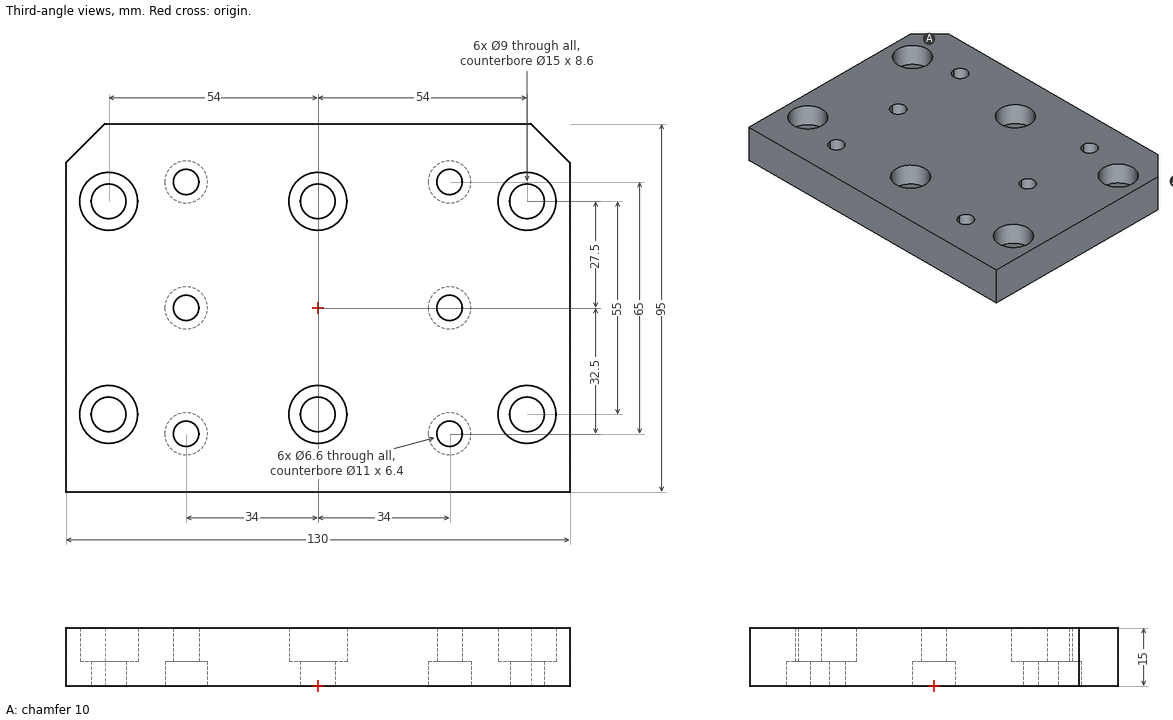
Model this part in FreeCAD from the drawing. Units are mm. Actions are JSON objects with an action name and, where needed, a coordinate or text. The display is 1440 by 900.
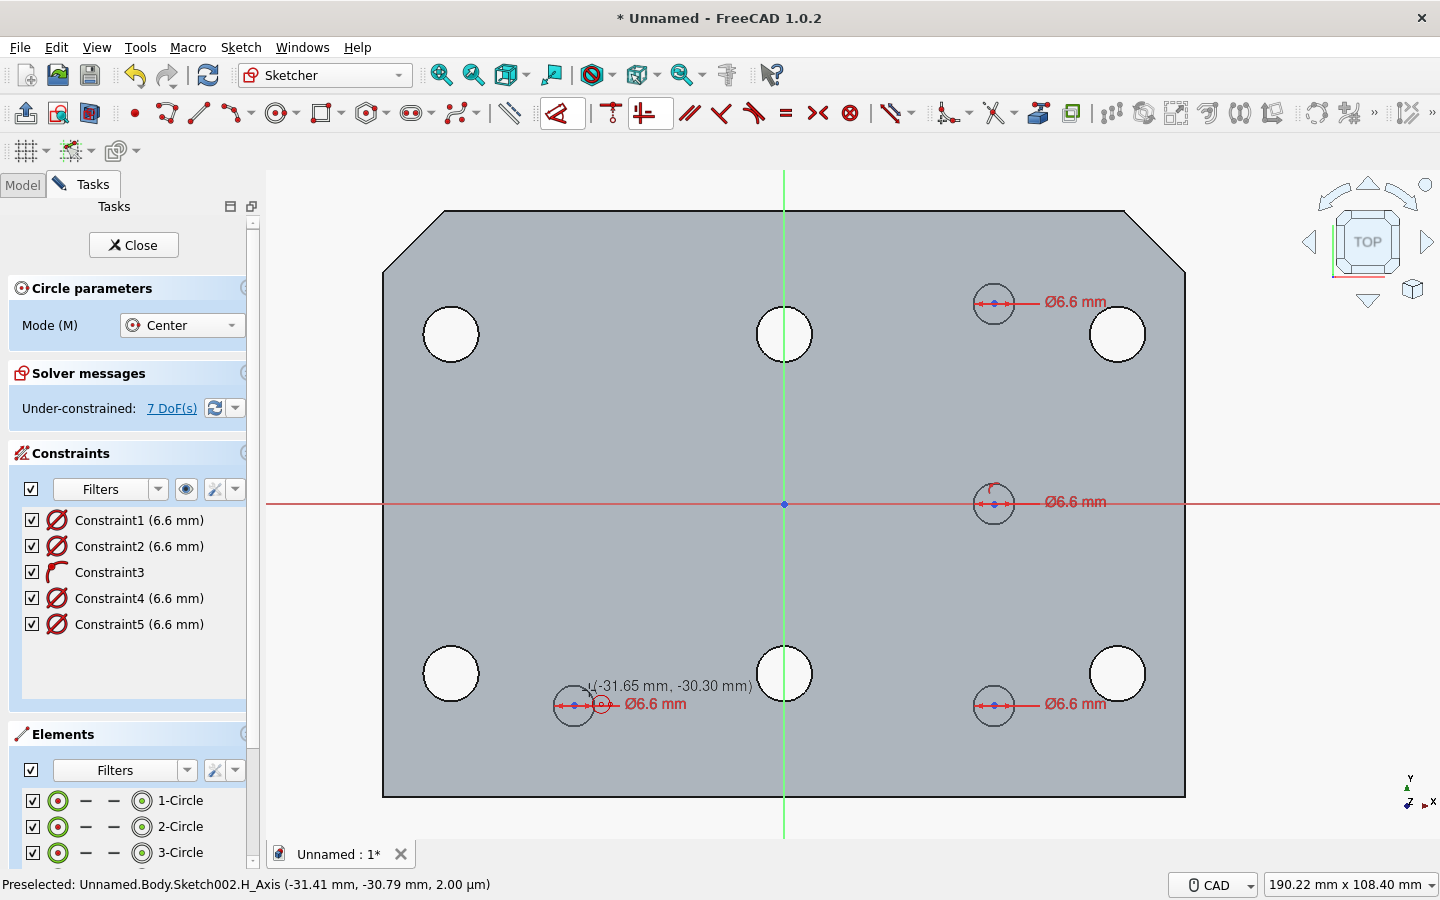
{"action": "left_click", "coordinate": [574, 504]}
{"action": "mouse_move", "coordinate": [589, 490]}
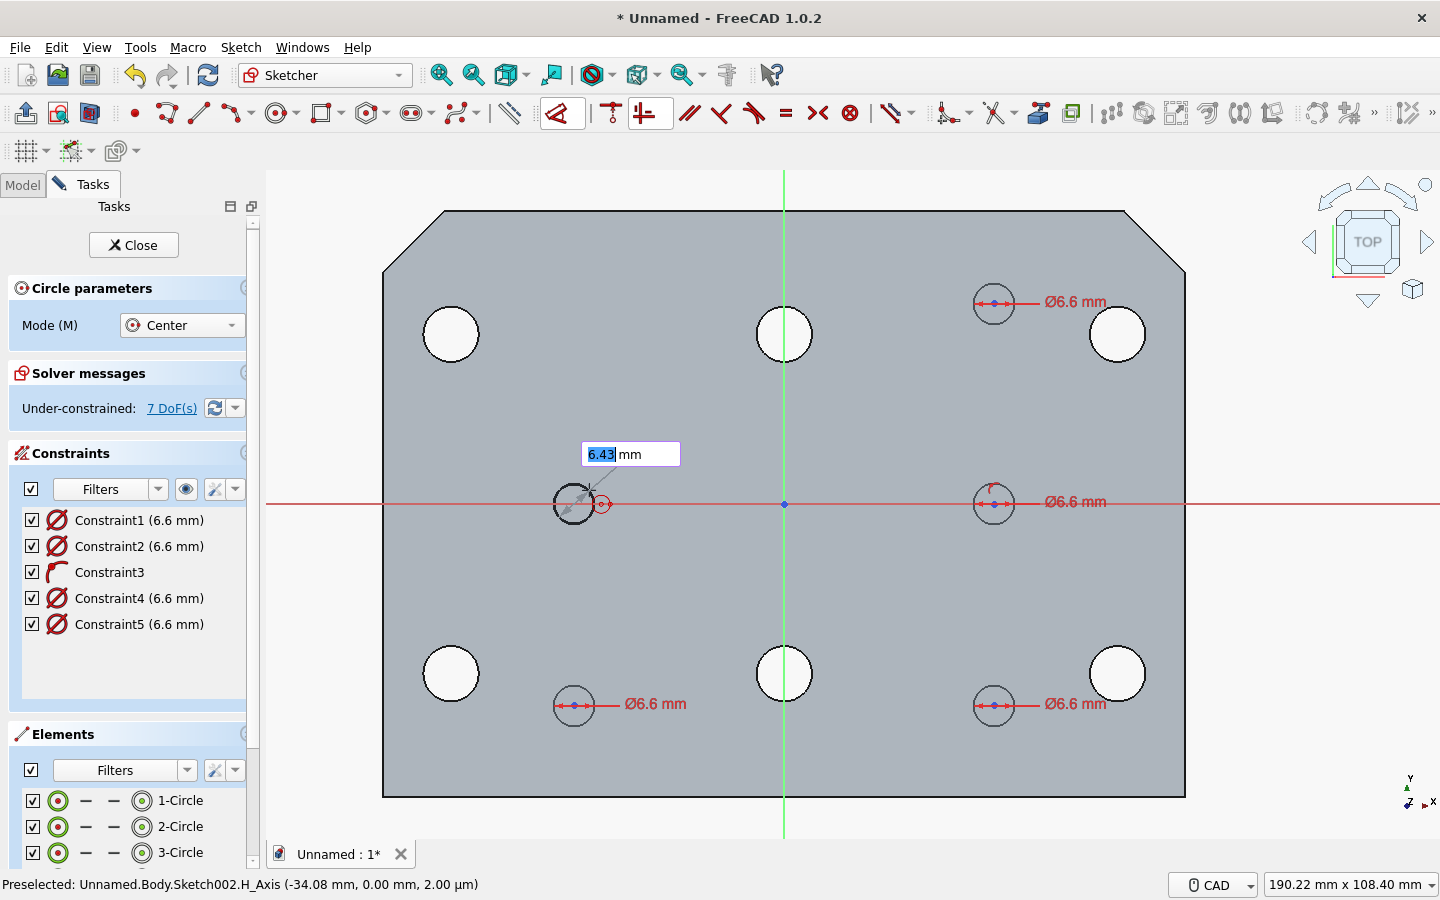
{"action": "type", "text": "6.6"}
{"action": "key", "text": "Return"}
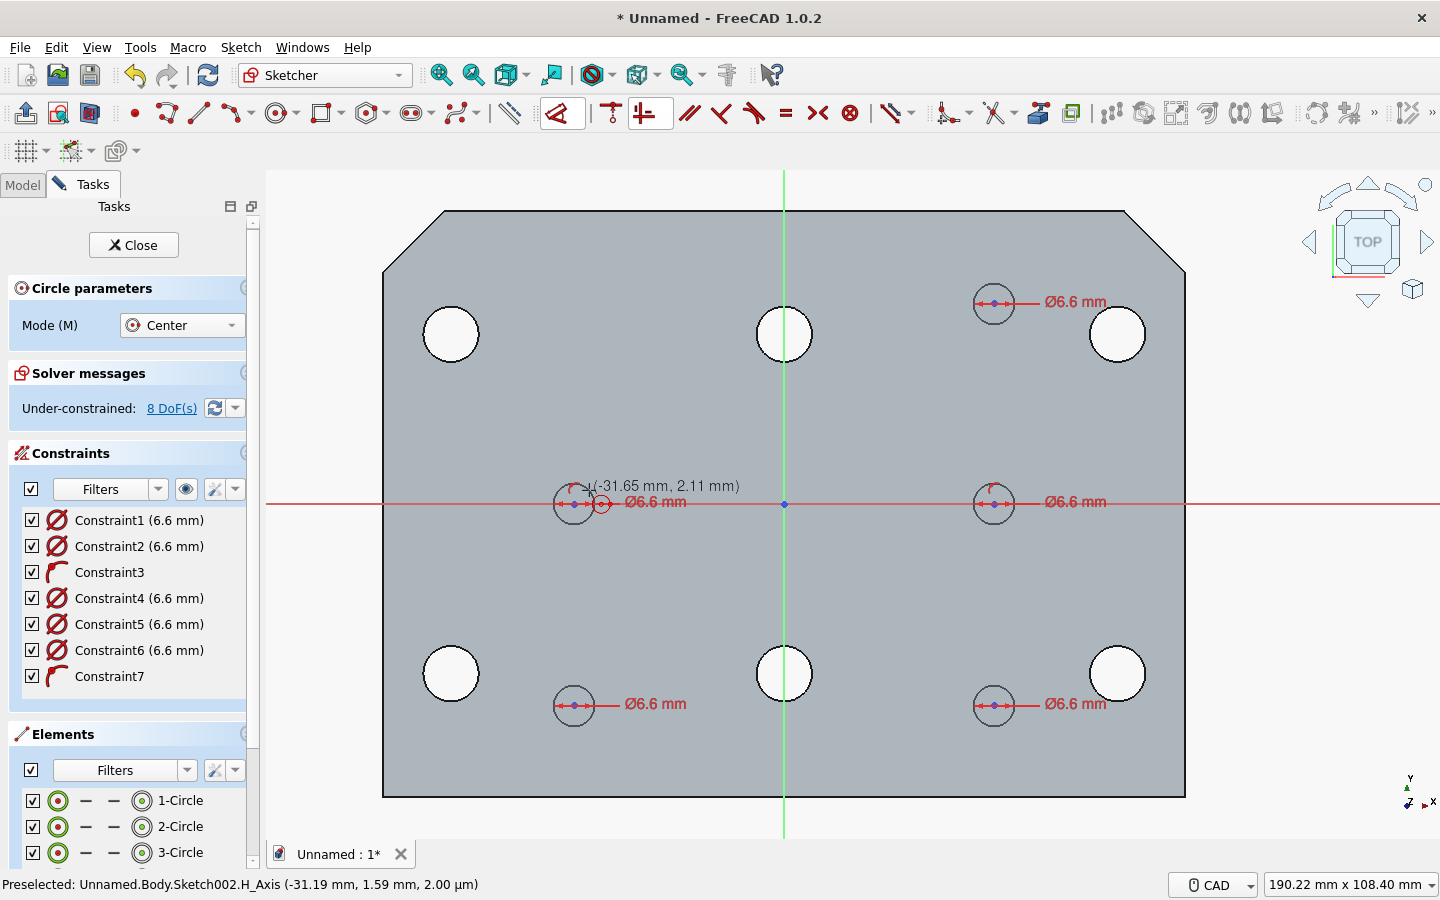
{"action": "left_click", "coordinate": [574, 303]}
{"action": "mouse_move", "coordinate": [589, 289]}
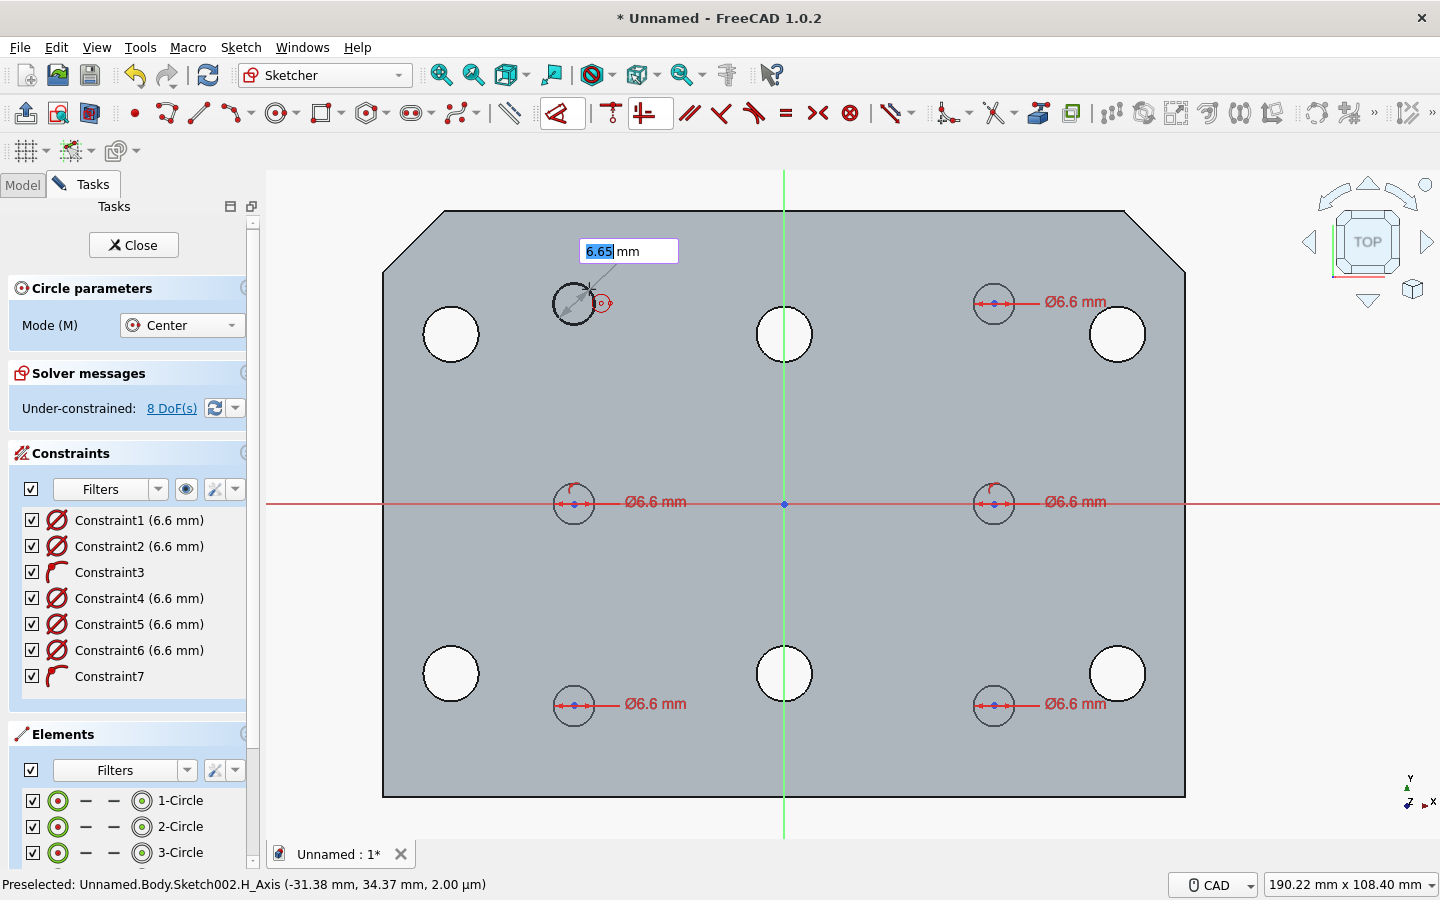
{"action": "type", "text": "6.6"}
{"action": "key", "text": "Return"}
{"action": "key", "text": "Escape"}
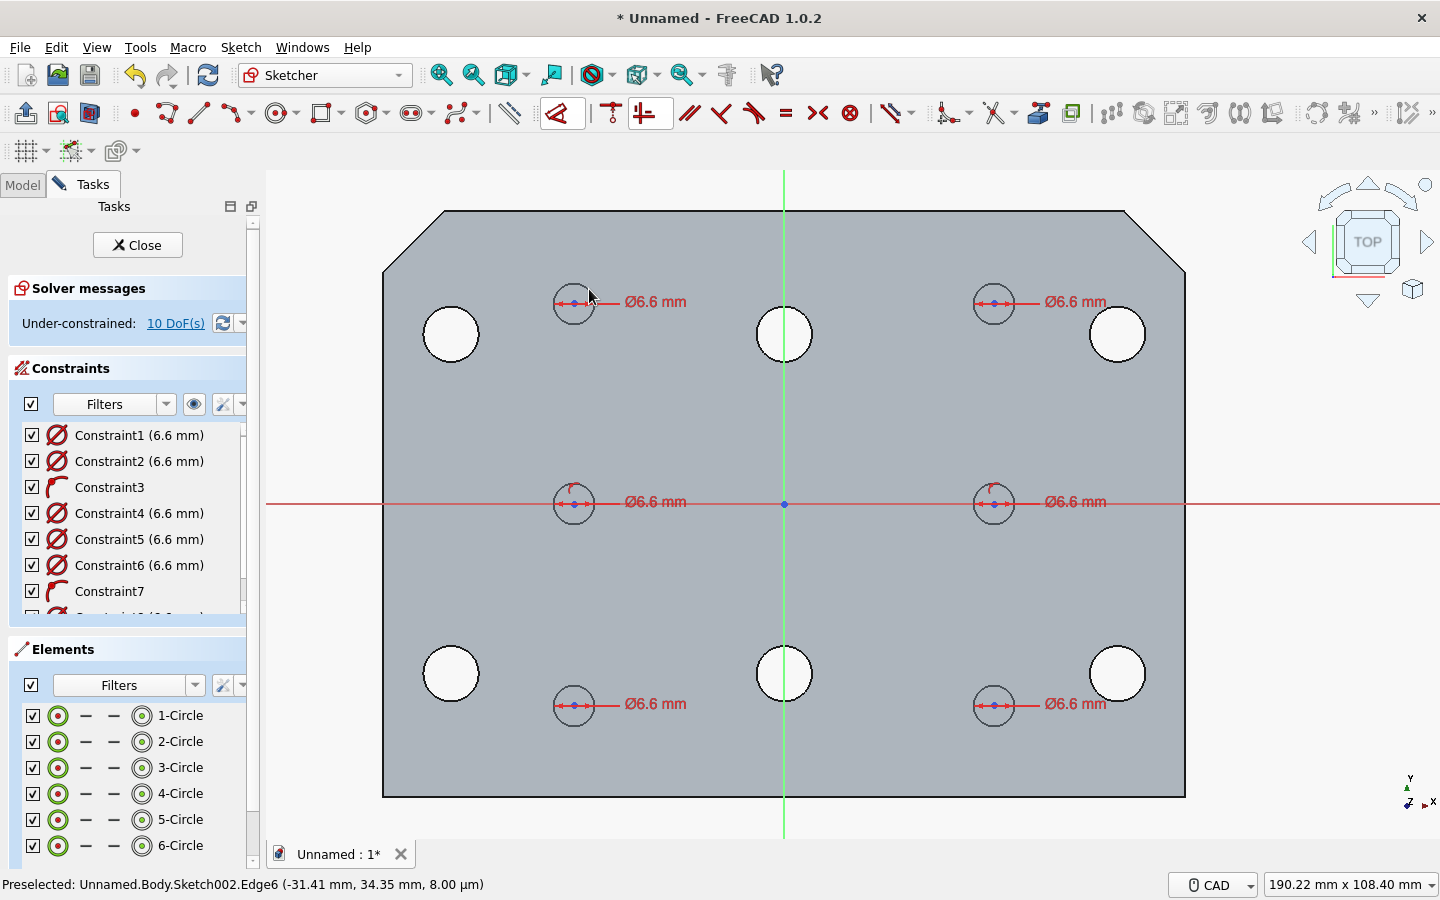
{"action": "left_click", "coordinate": [994, 706]}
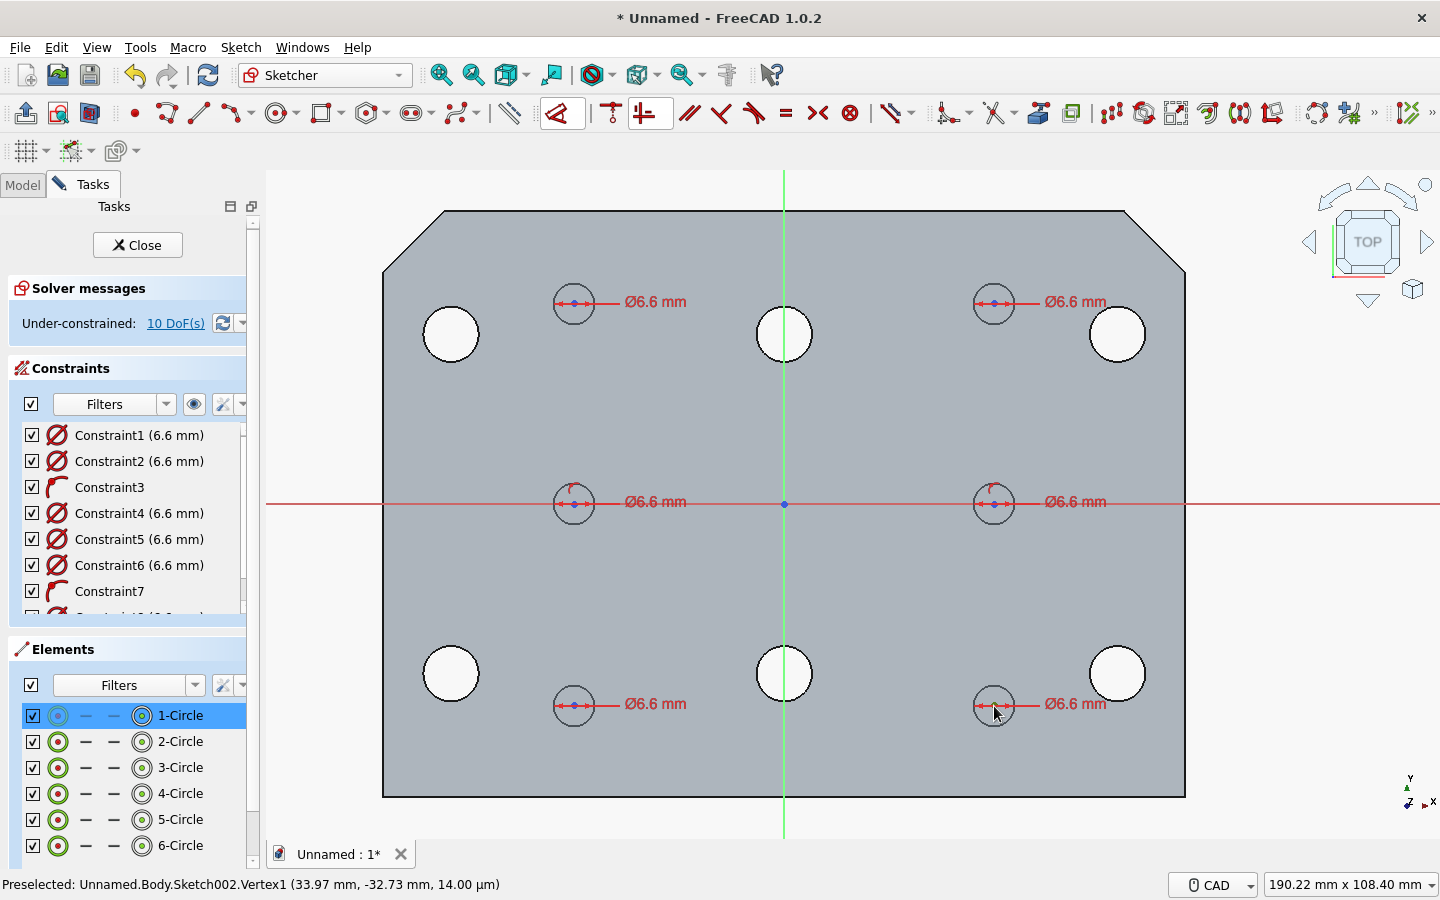
{"action": "left_click", "coordinate": [994, 504]}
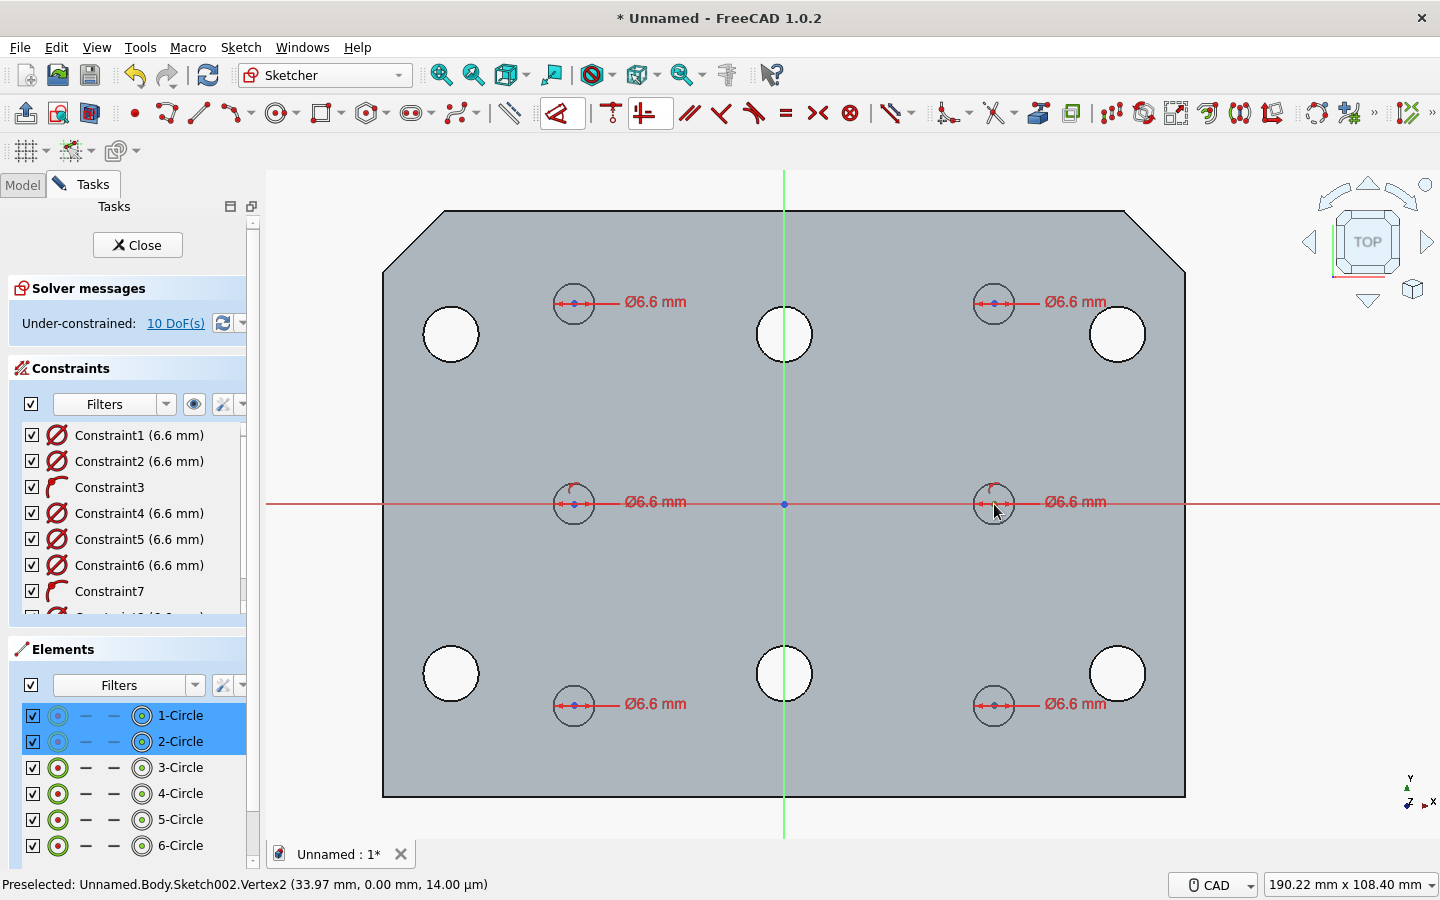
{"action": "key", "text": "v"}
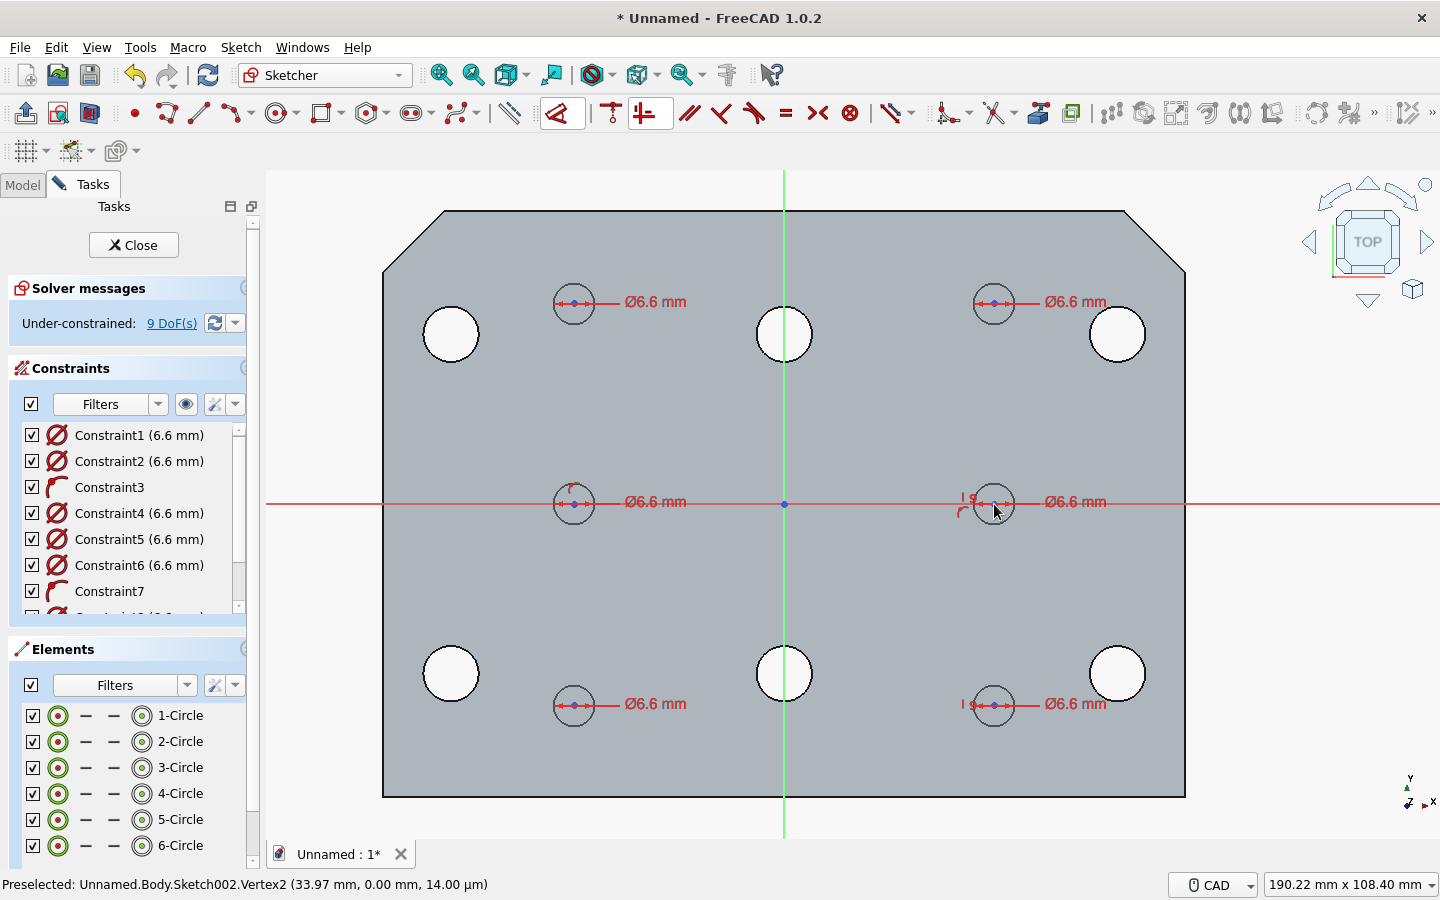
{"action": "left_click", "coordinate": [994, 504]}